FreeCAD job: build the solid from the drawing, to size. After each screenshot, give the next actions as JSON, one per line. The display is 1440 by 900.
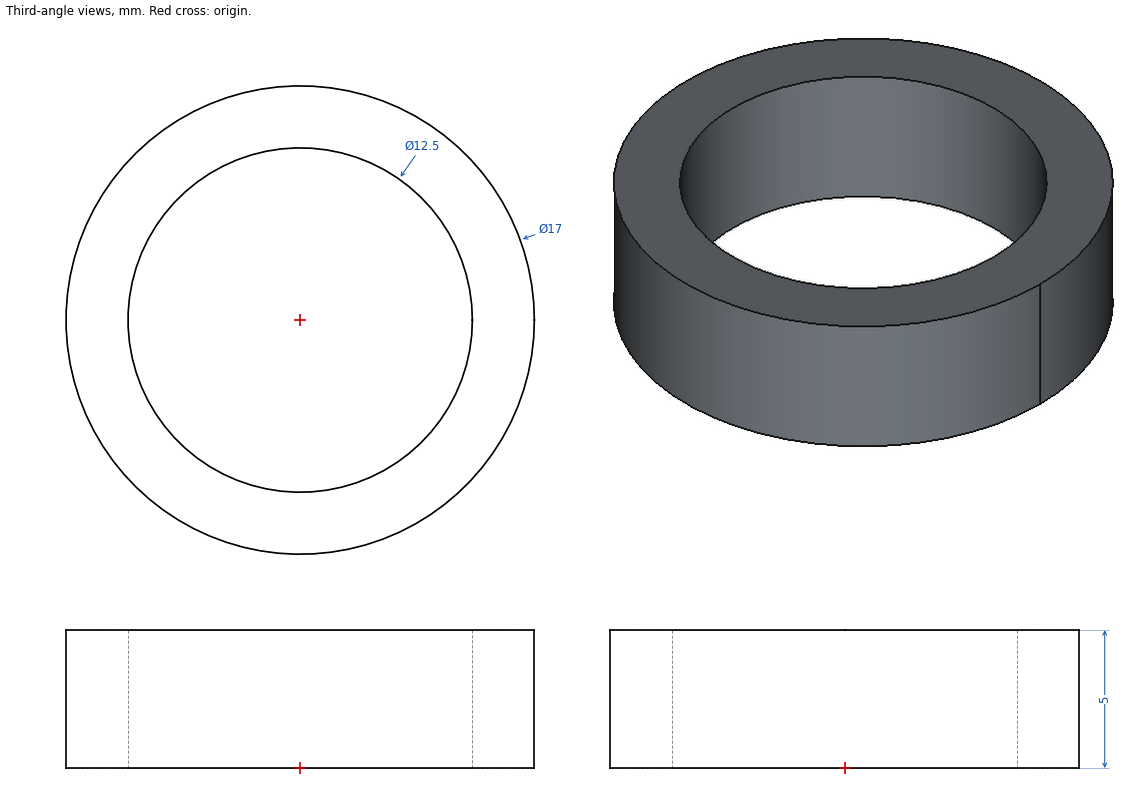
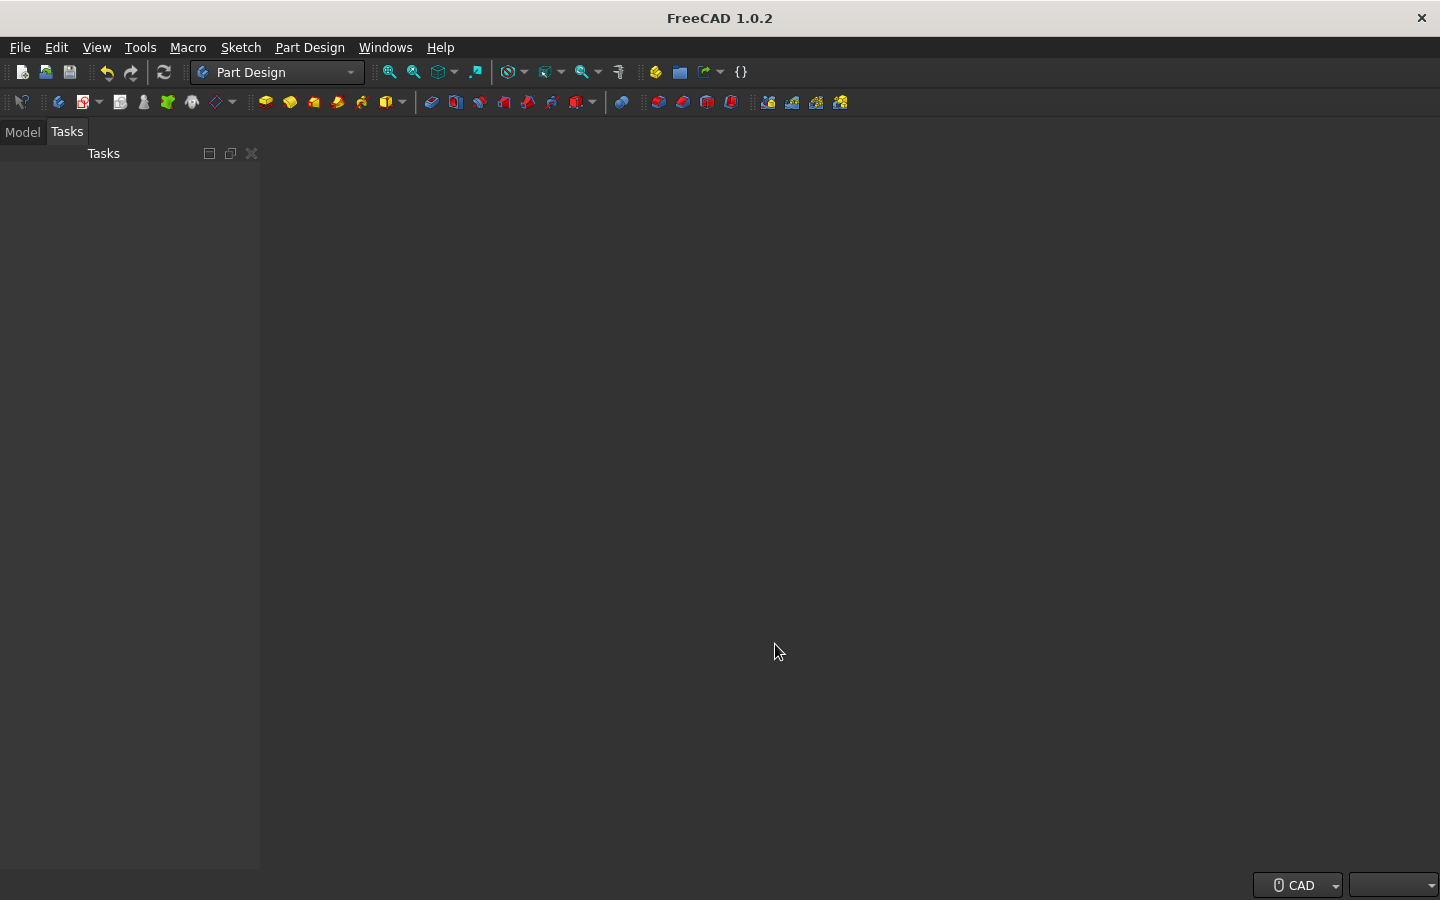
{"action": "key", "text": "ctrl+n"}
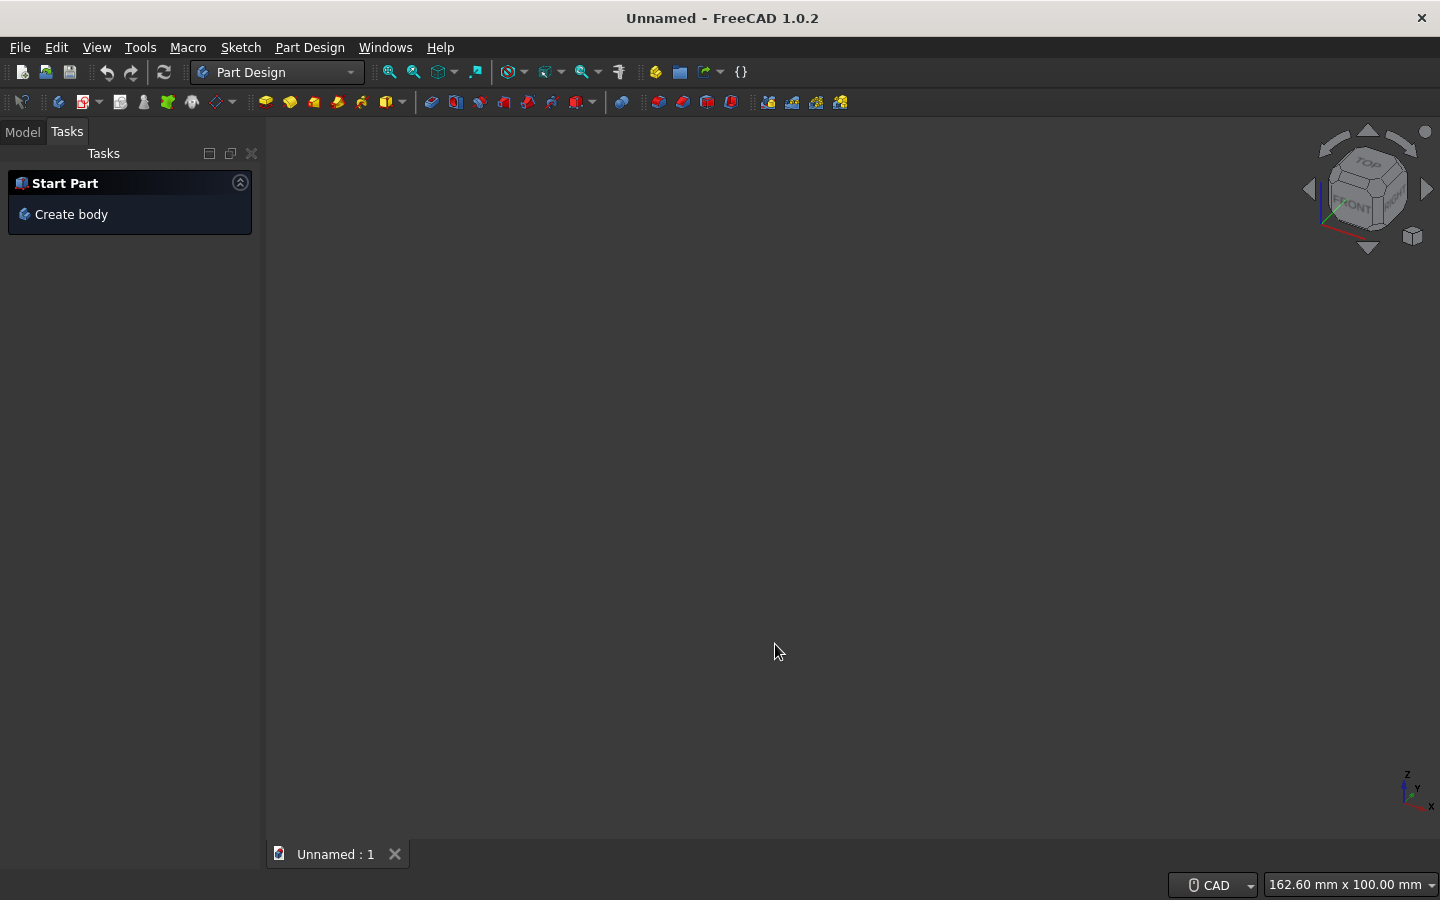
{"action": "left_click", "coordinate": [84, 102]}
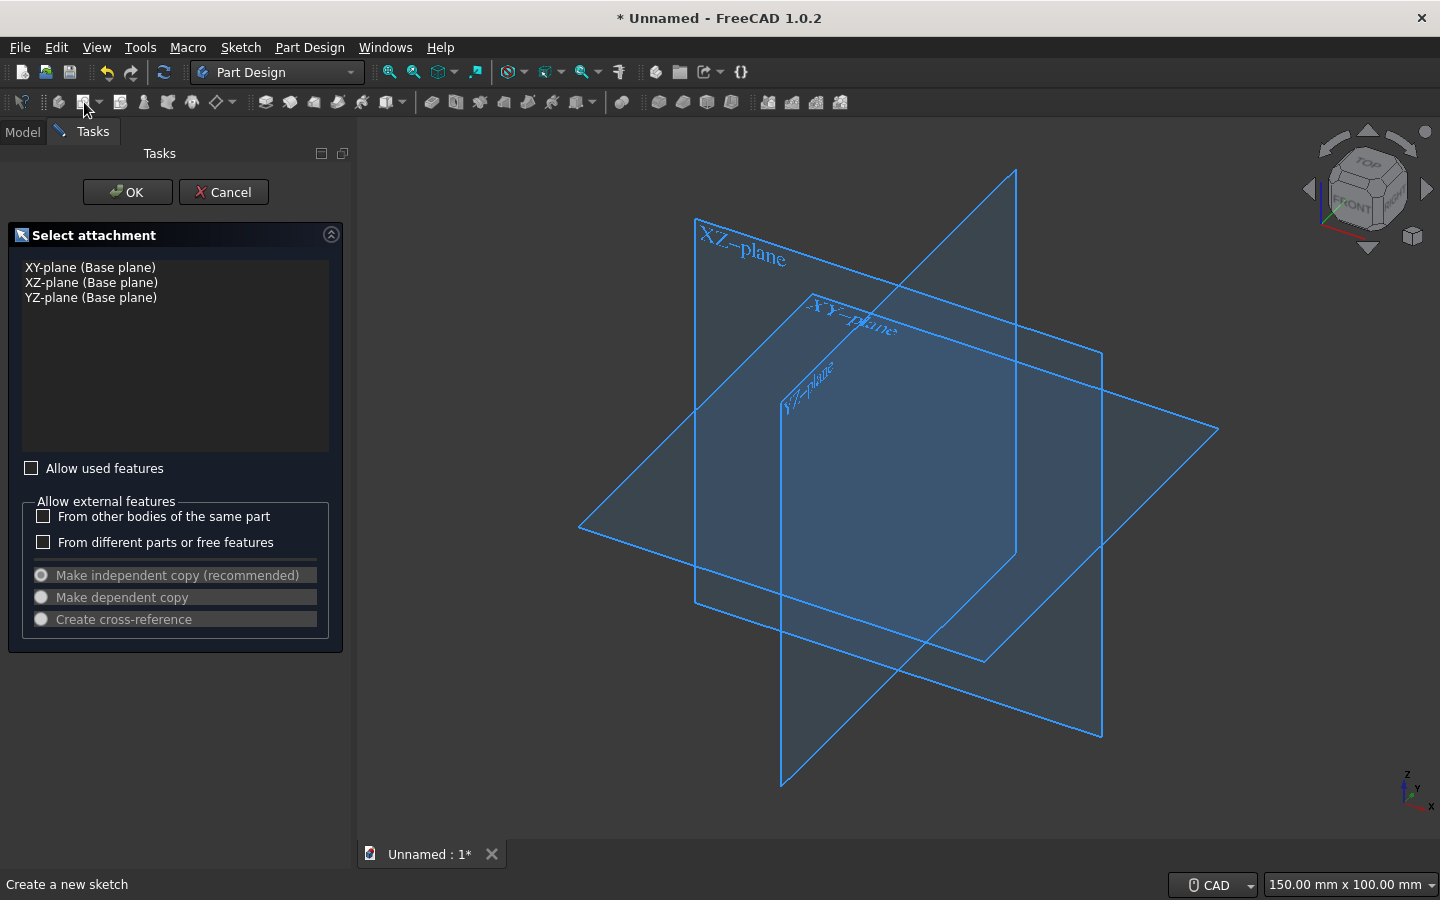
{"action": "left_click", "coordinate": [82, 268]}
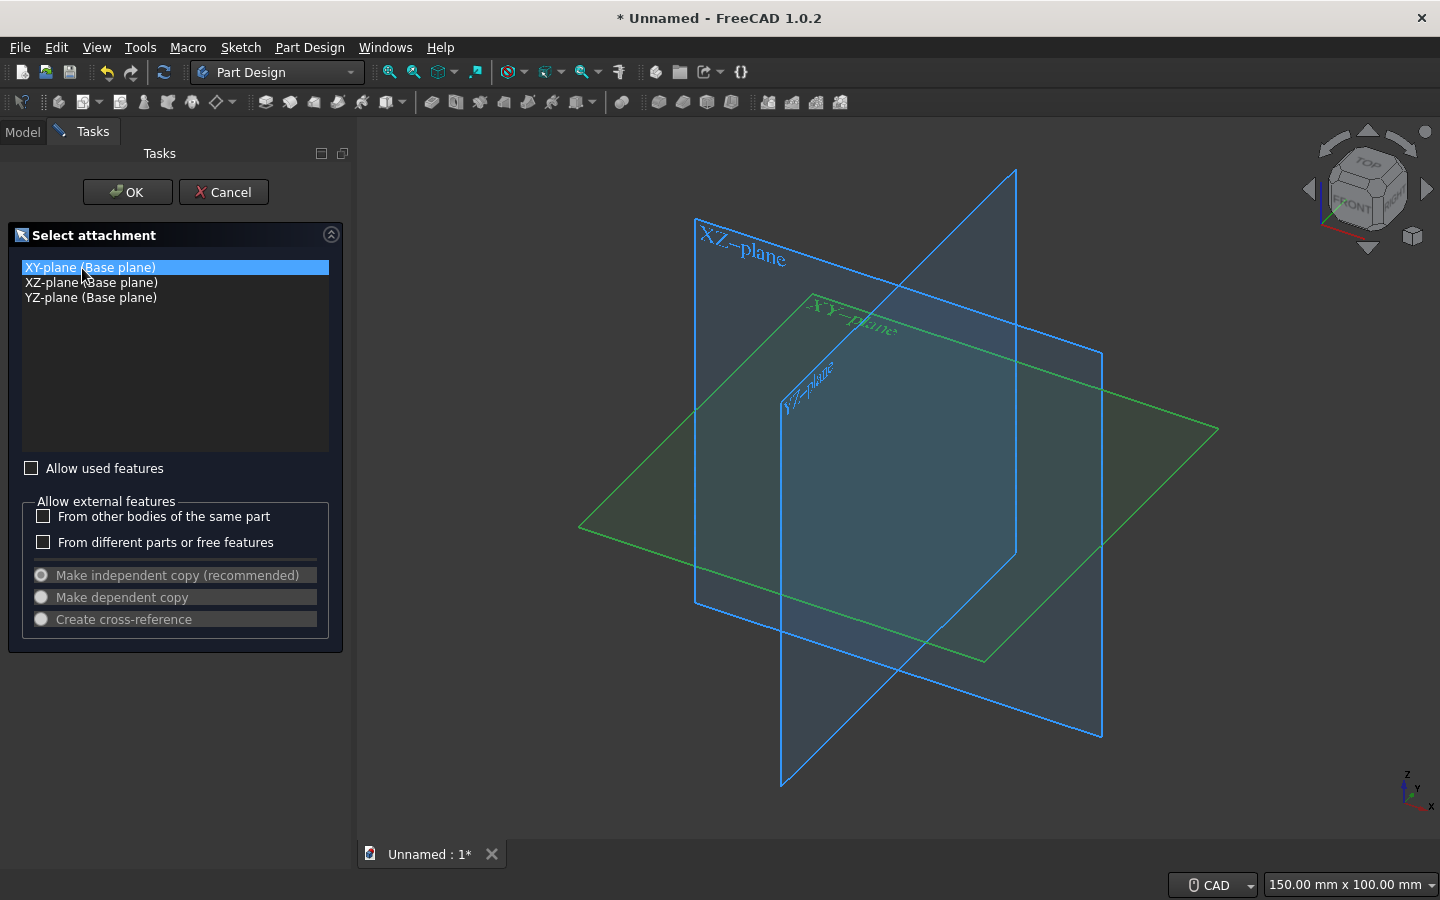
{"action": "left_click", "coordinate": [128, 192]}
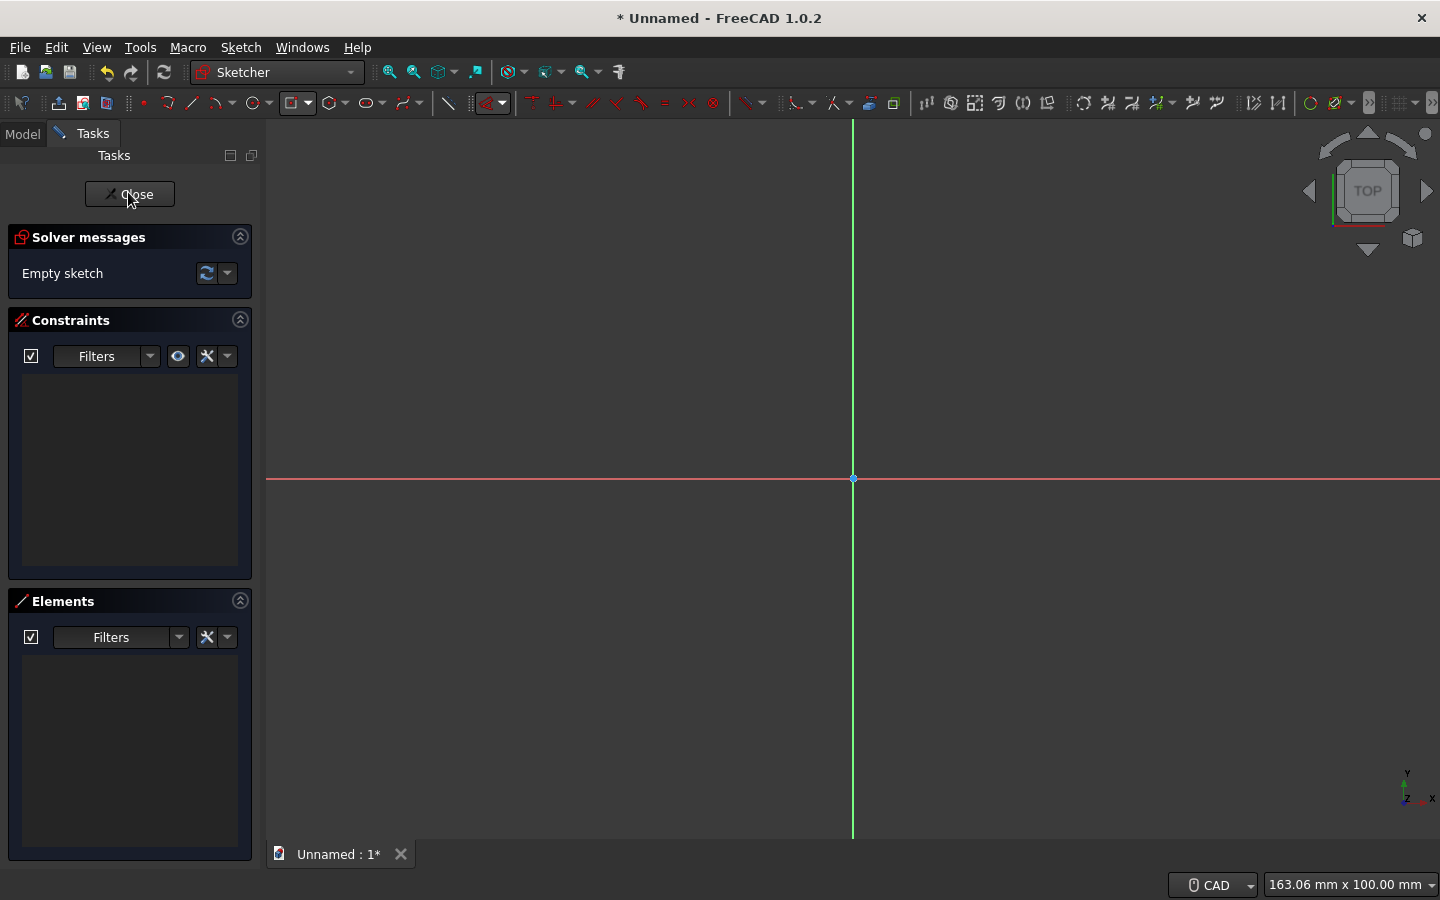
{"action": "scroll", "coordinate": [875, 479], "scroll_direction": "up", "scroll_amount": 7}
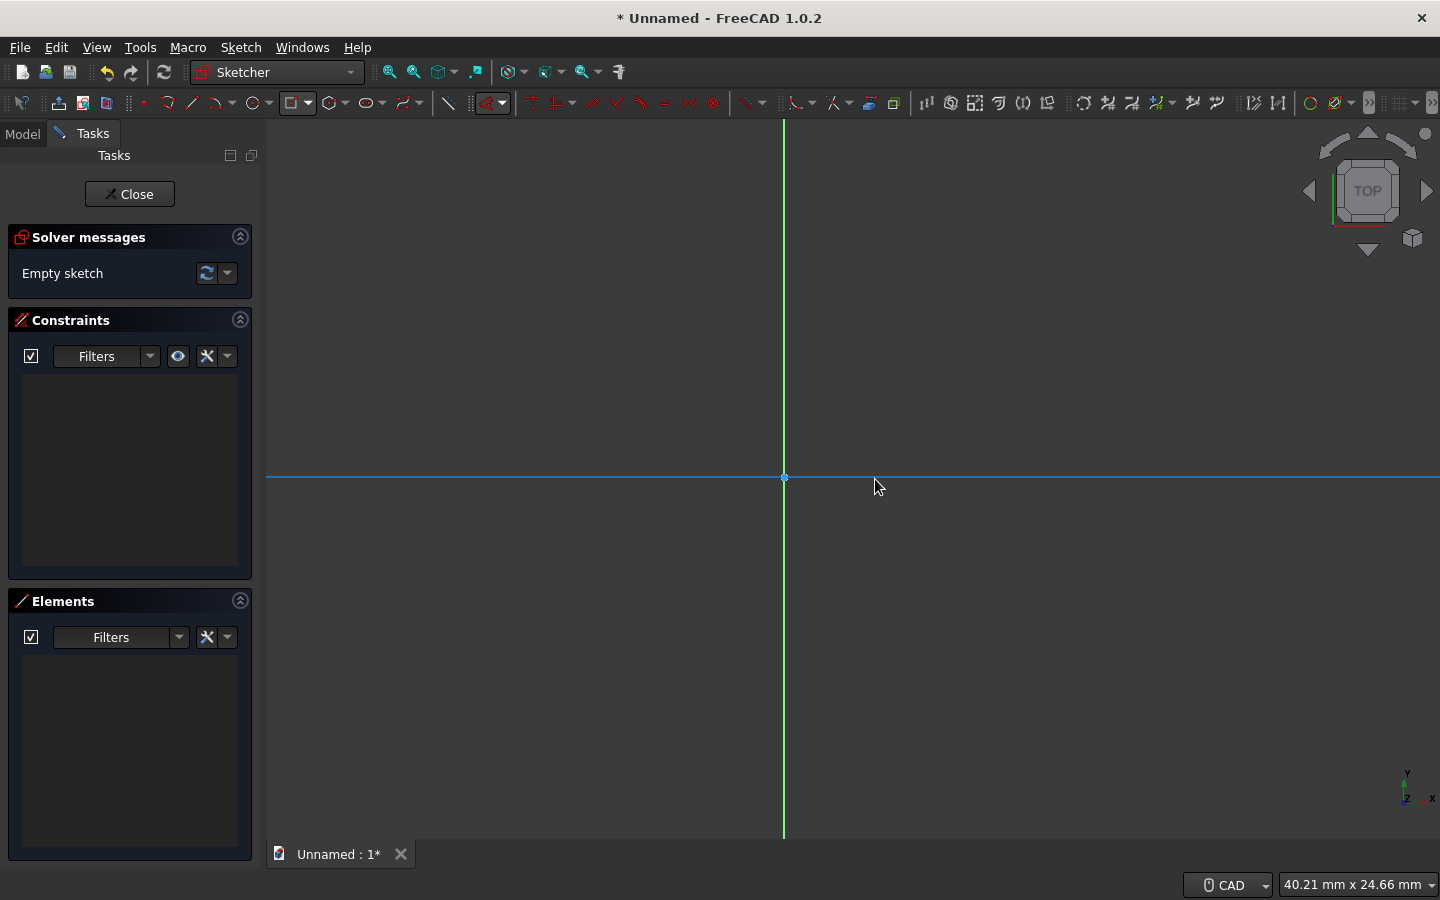
{"action": "key", "text": "g c"}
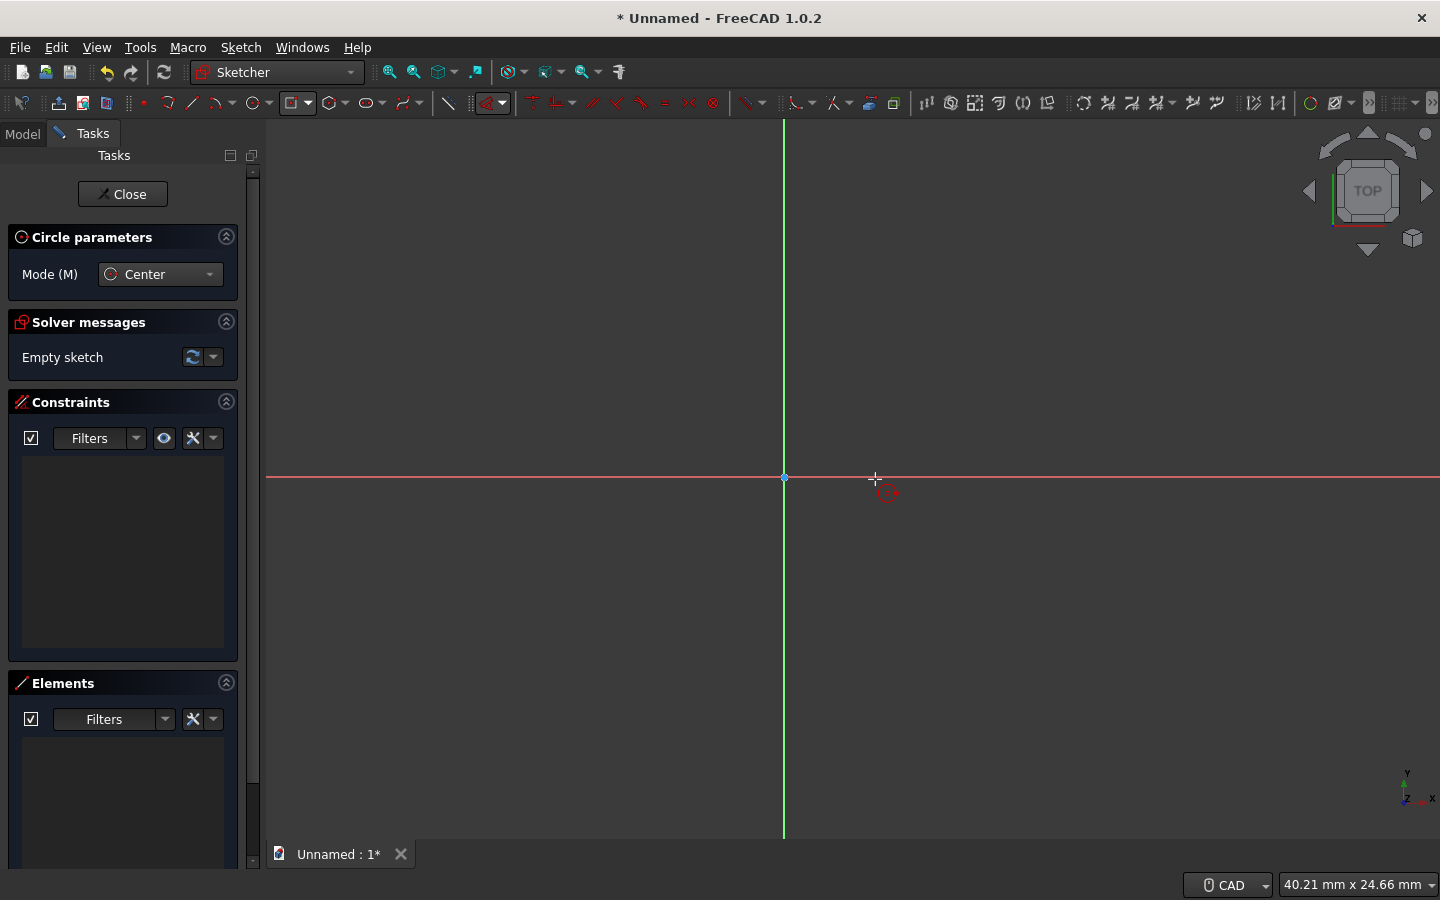
{"action": "left_click", "coordinate": [784, 477]}
{"action": "left_click", "coordinate": [960, 302]}